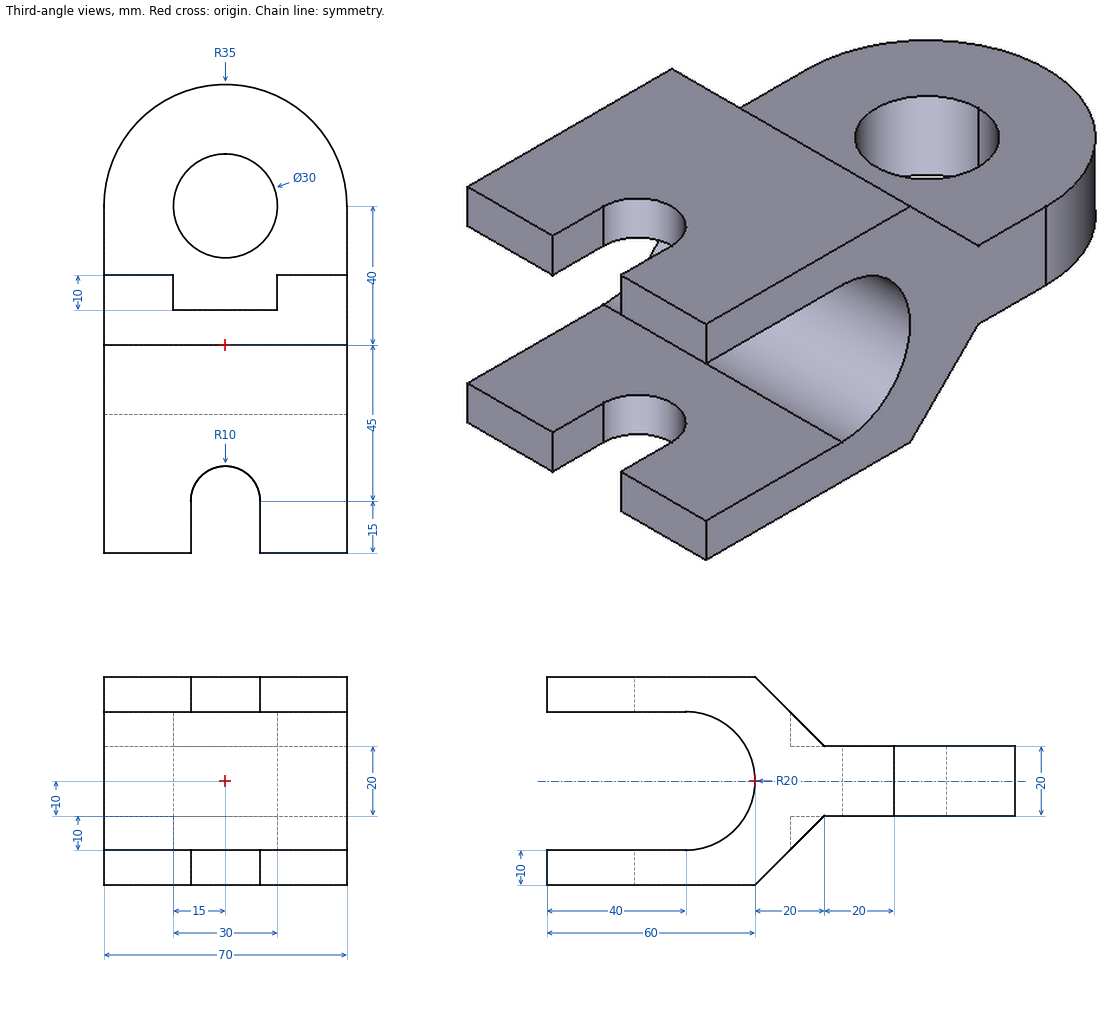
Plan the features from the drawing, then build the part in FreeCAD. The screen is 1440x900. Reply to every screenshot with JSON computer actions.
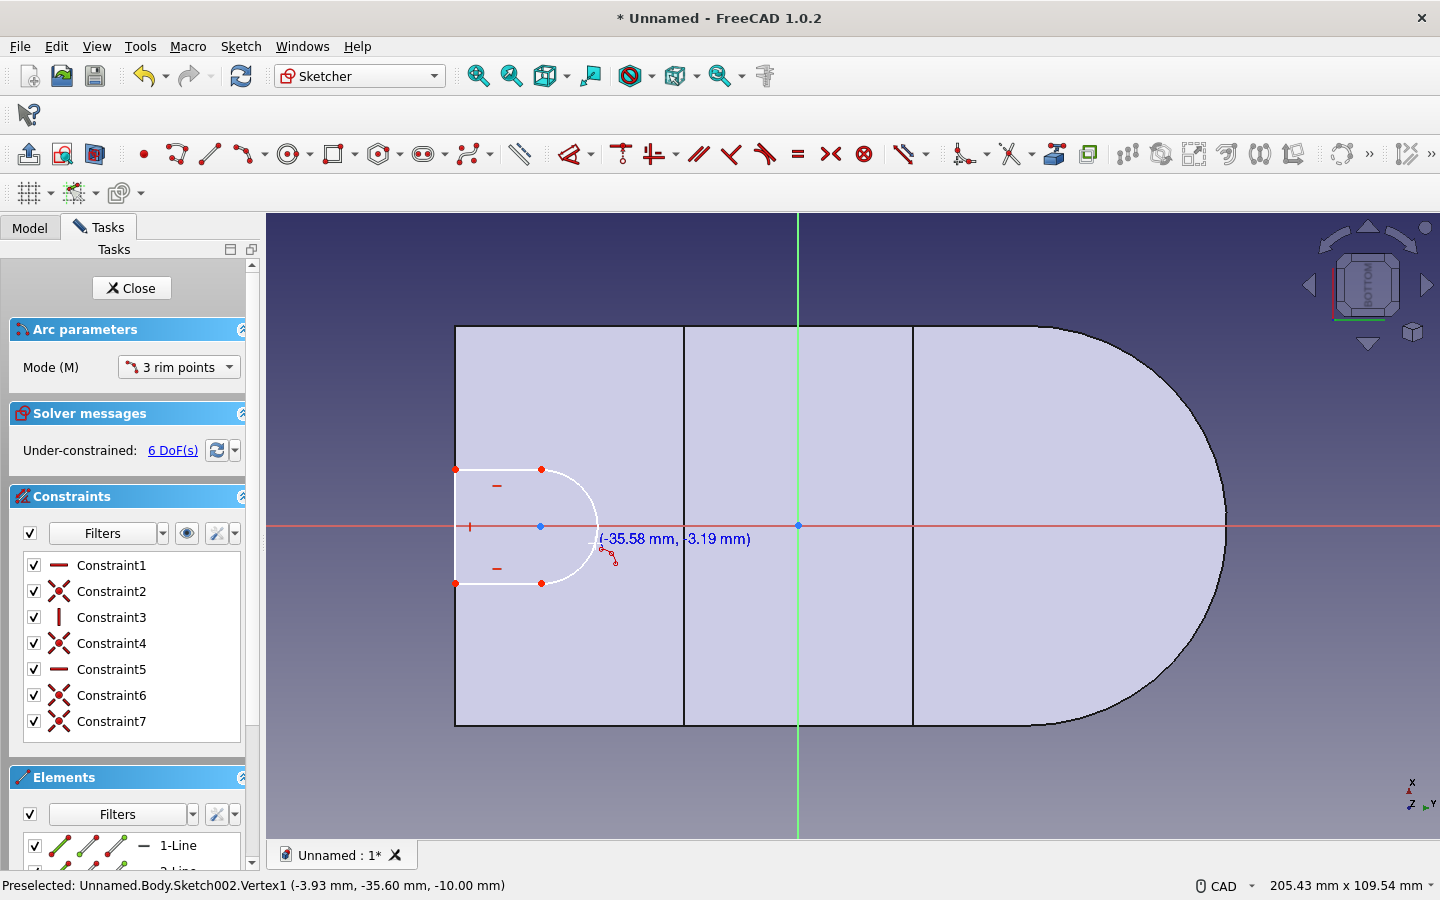
{"action": "key", "text": "g c"}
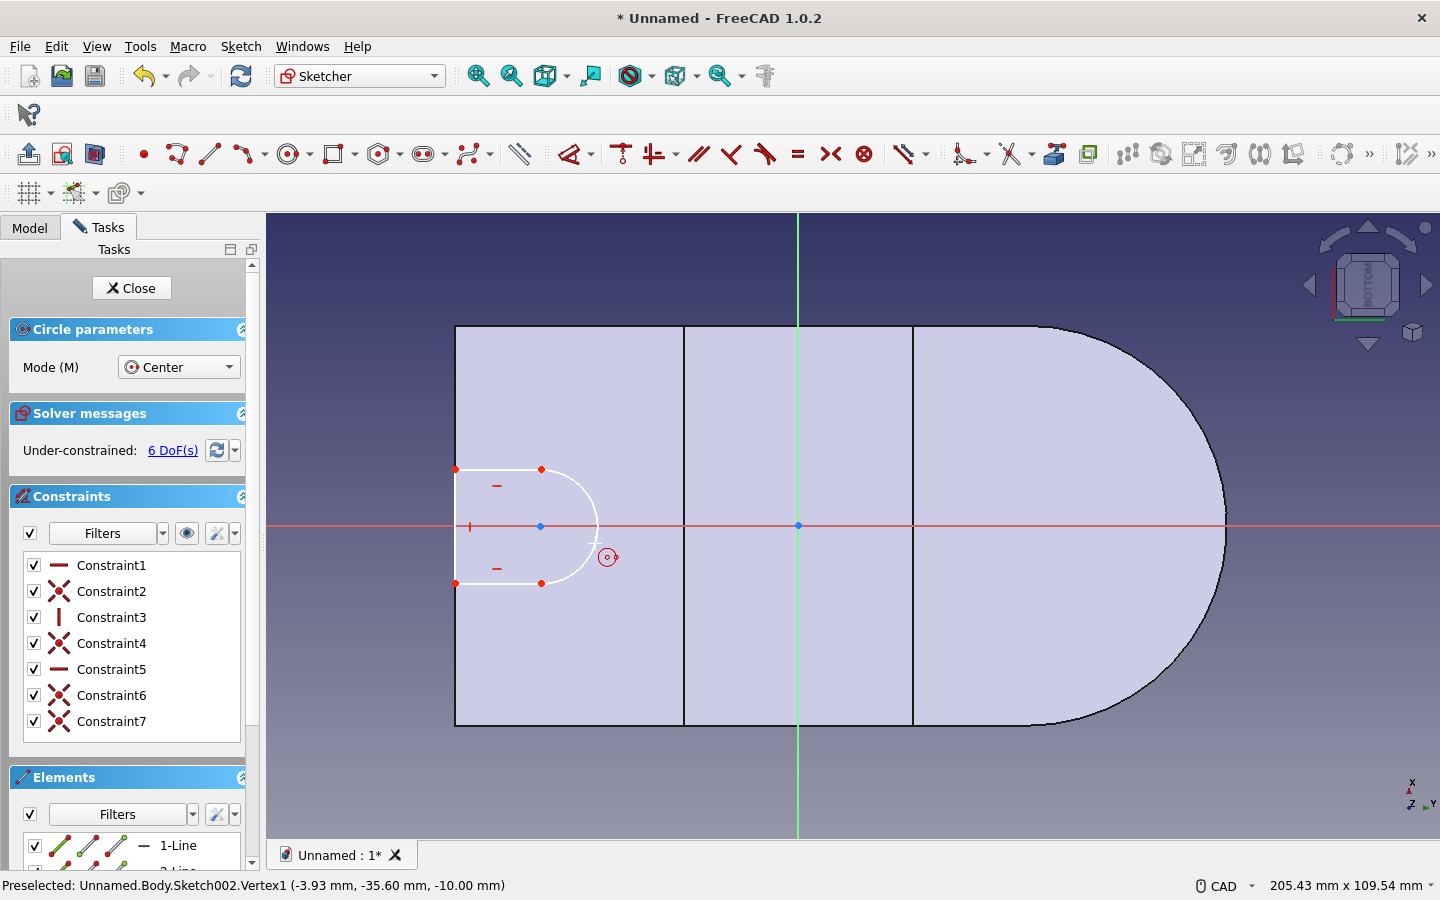
{"action": "left_click", "coordinate": [1027, 526]}
{"action": "left_click", "coordinate": [1088, 465]}
{"action": "key", "text": "Escape"}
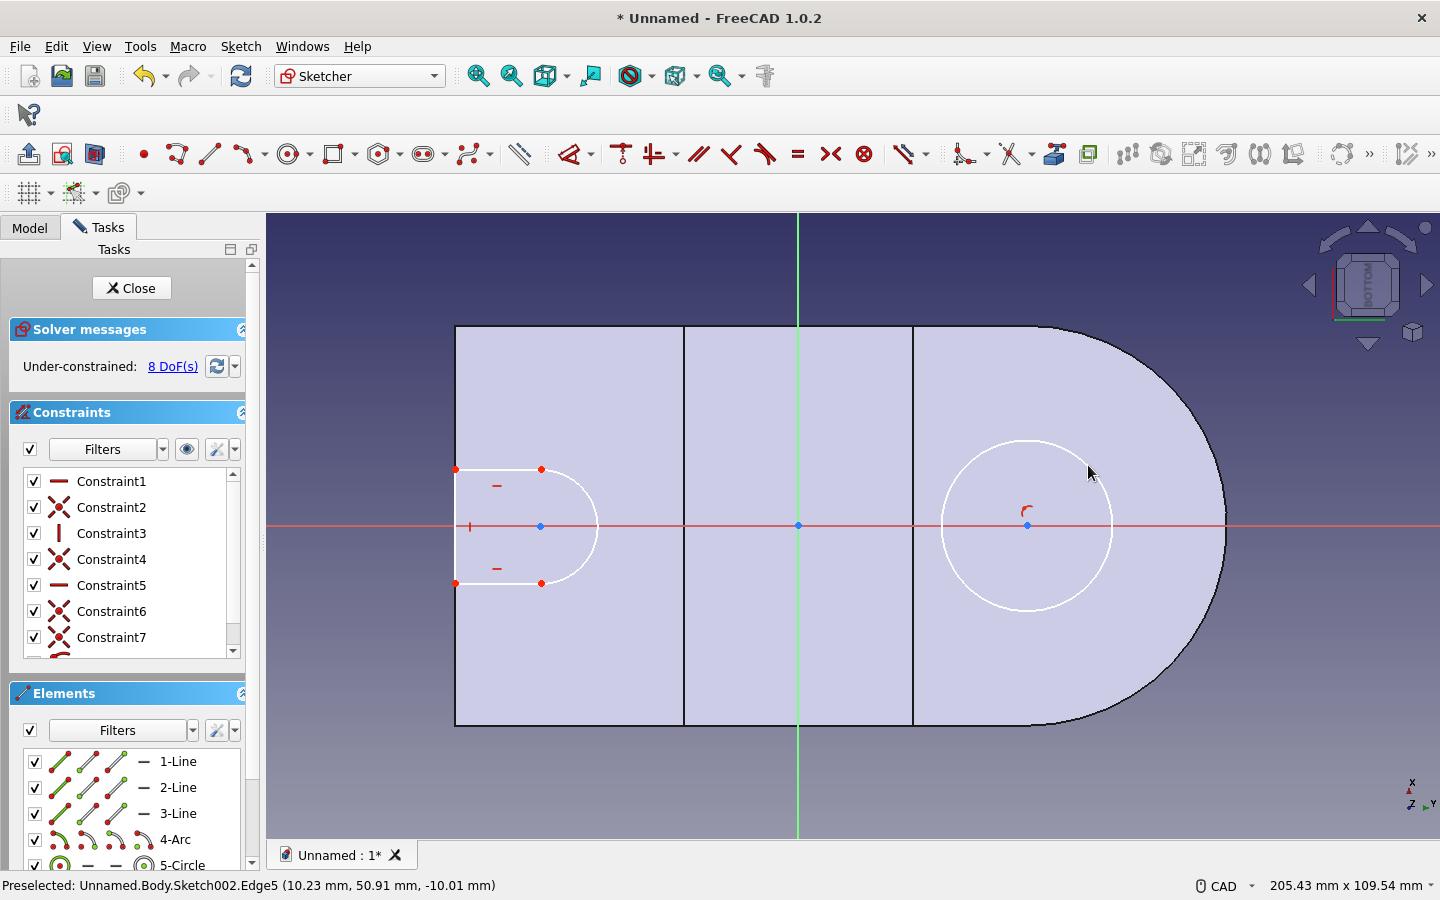
{"action": "left_click", "coordinate": [515, 470]}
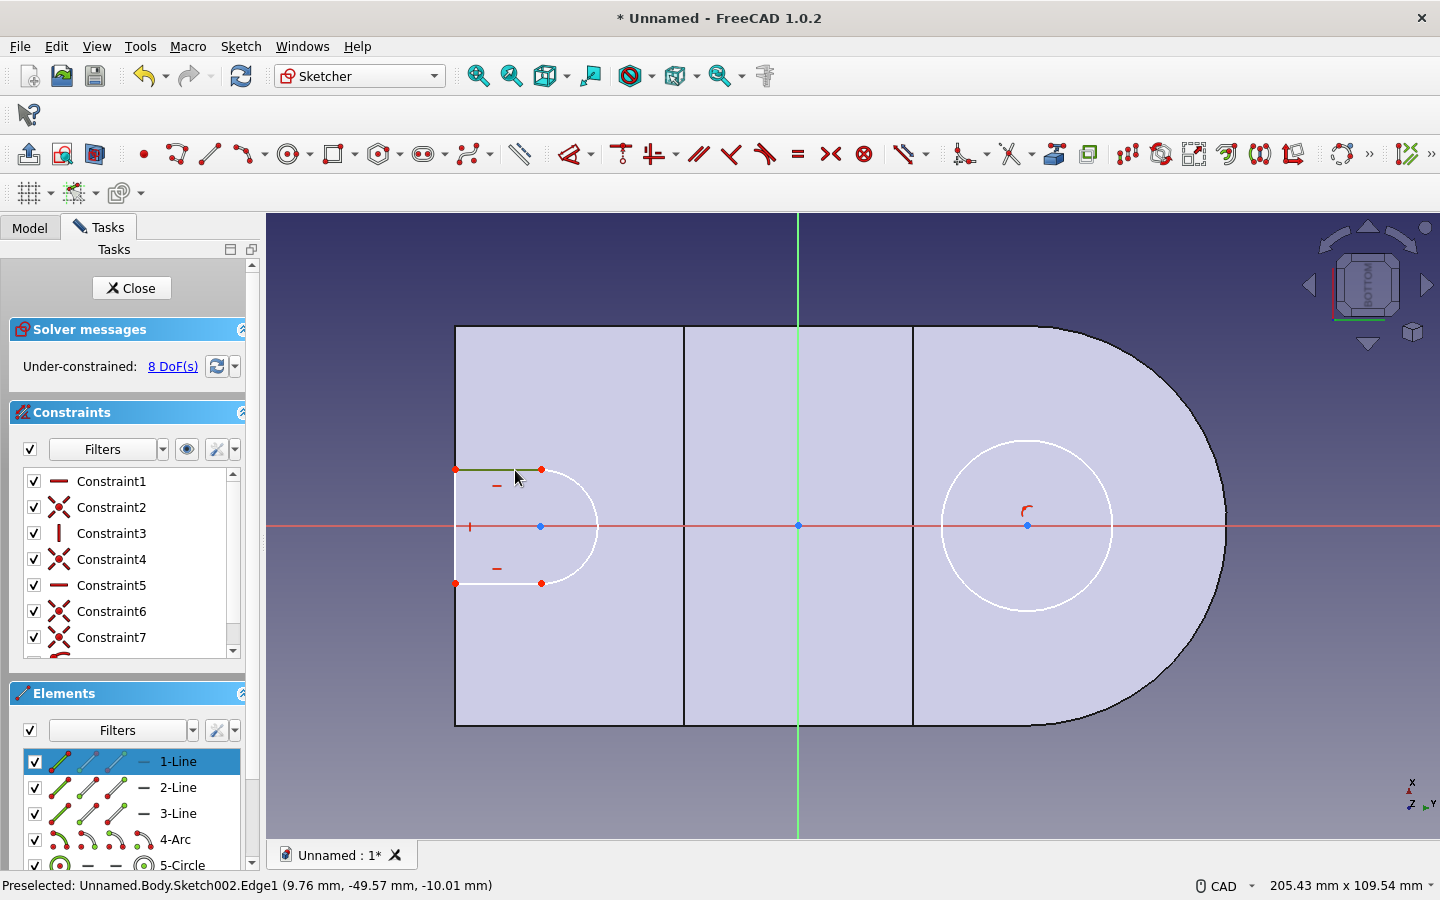
{"action": "left_click", "coordinate": [587, 560]}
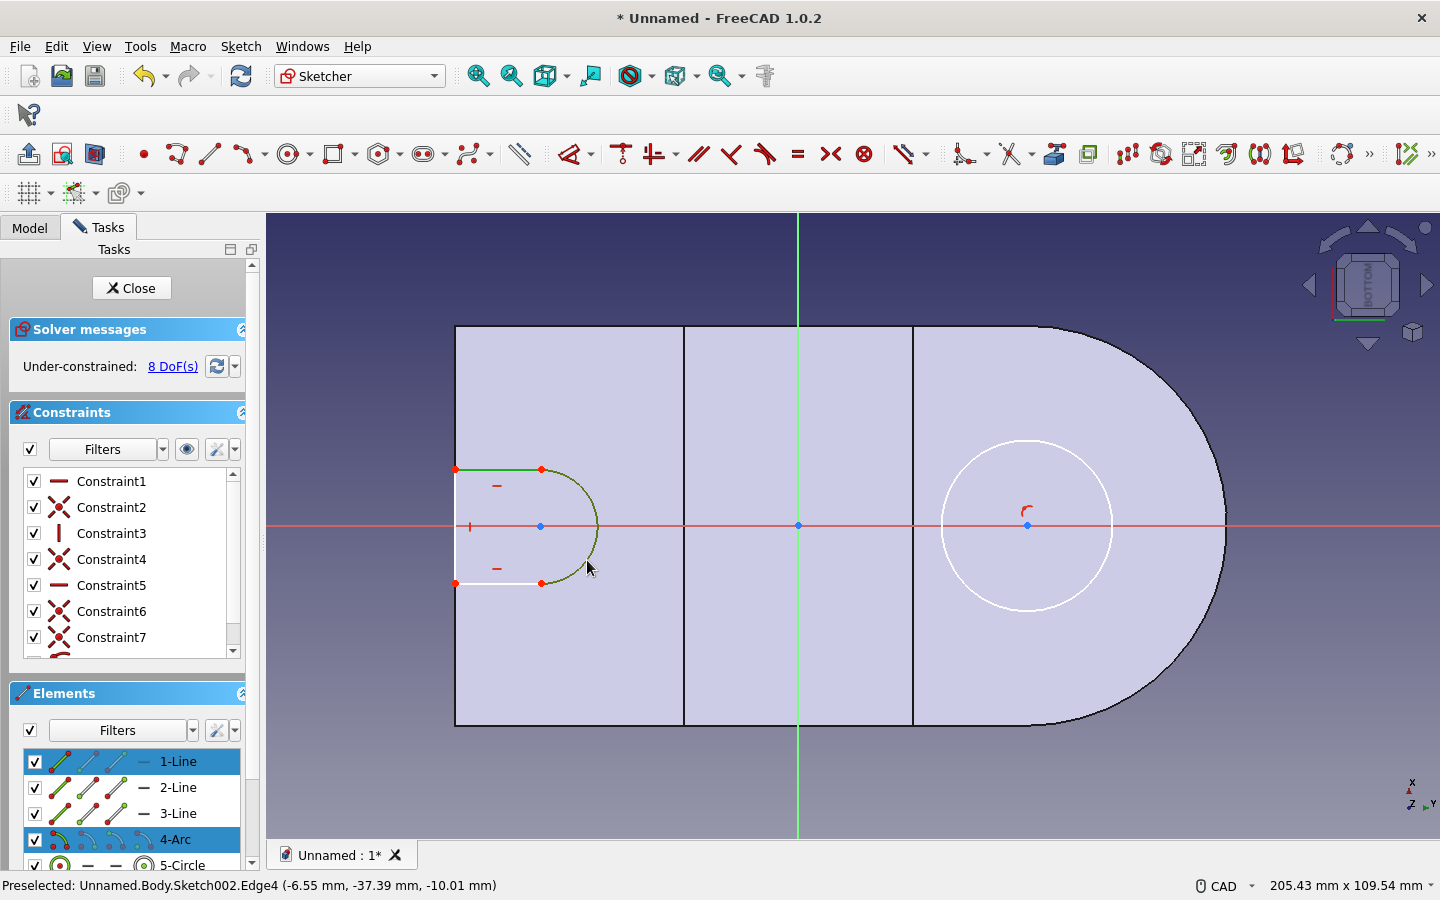
{"action": "left_click", "coordinate": [765, 154]}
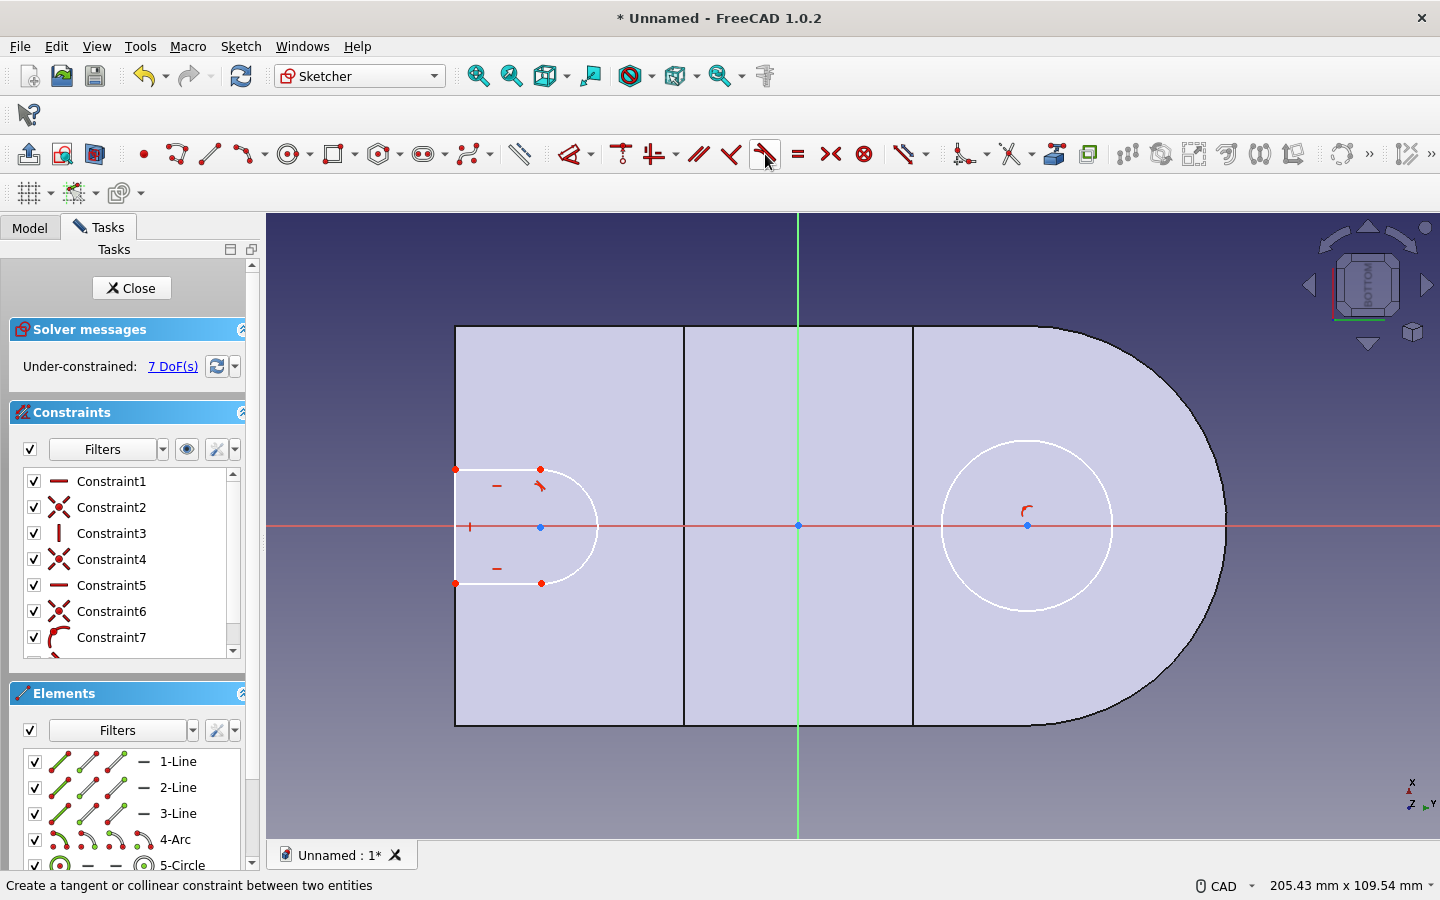
{"action": "left_click", "coordinate": [481, 584]}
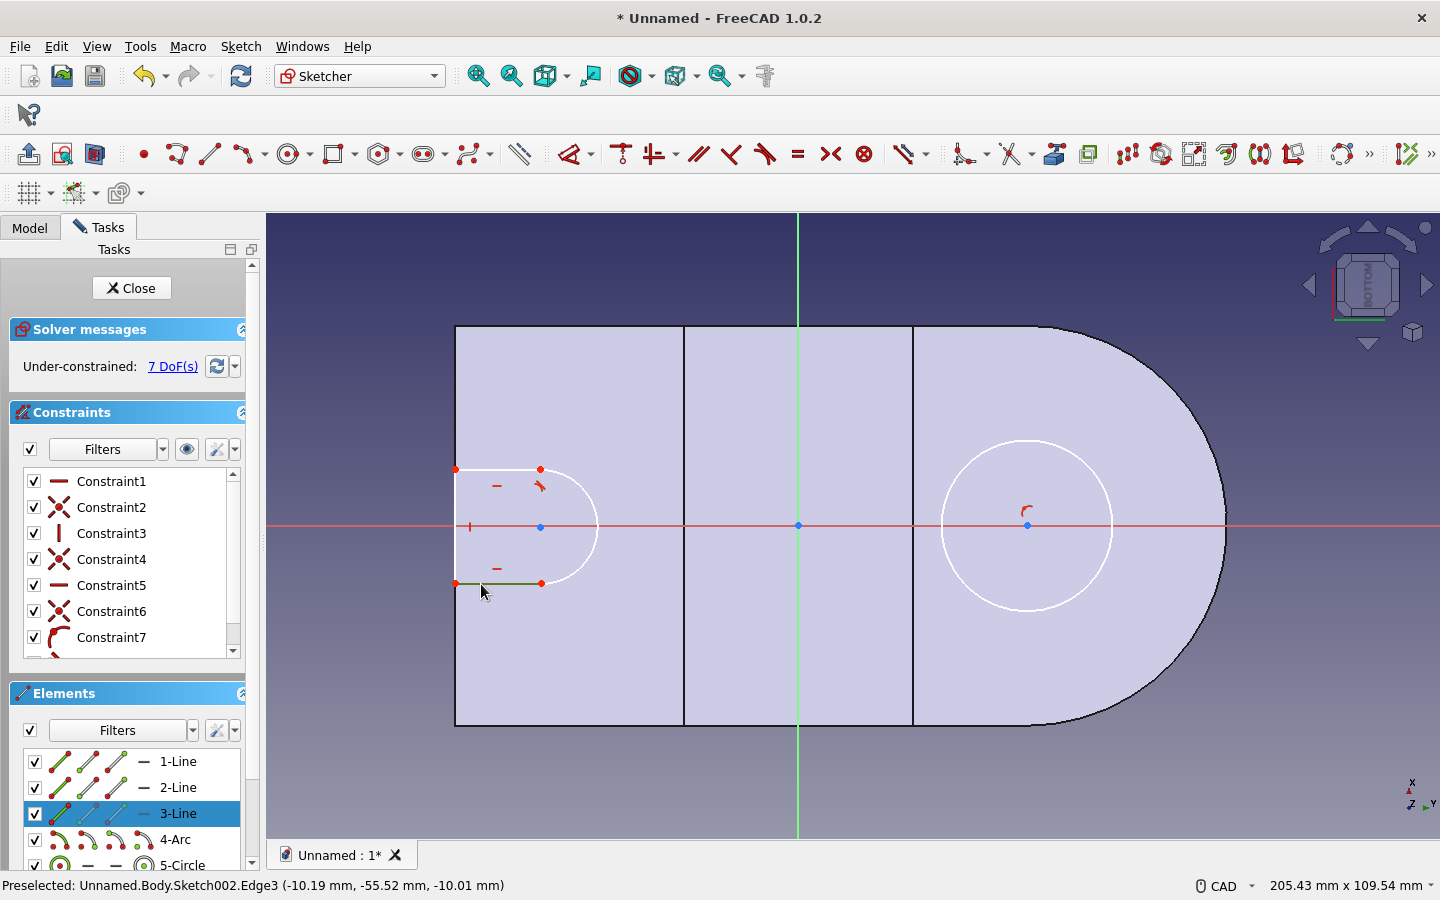
{"action": "left_click", "coordinate": [587, 560]}